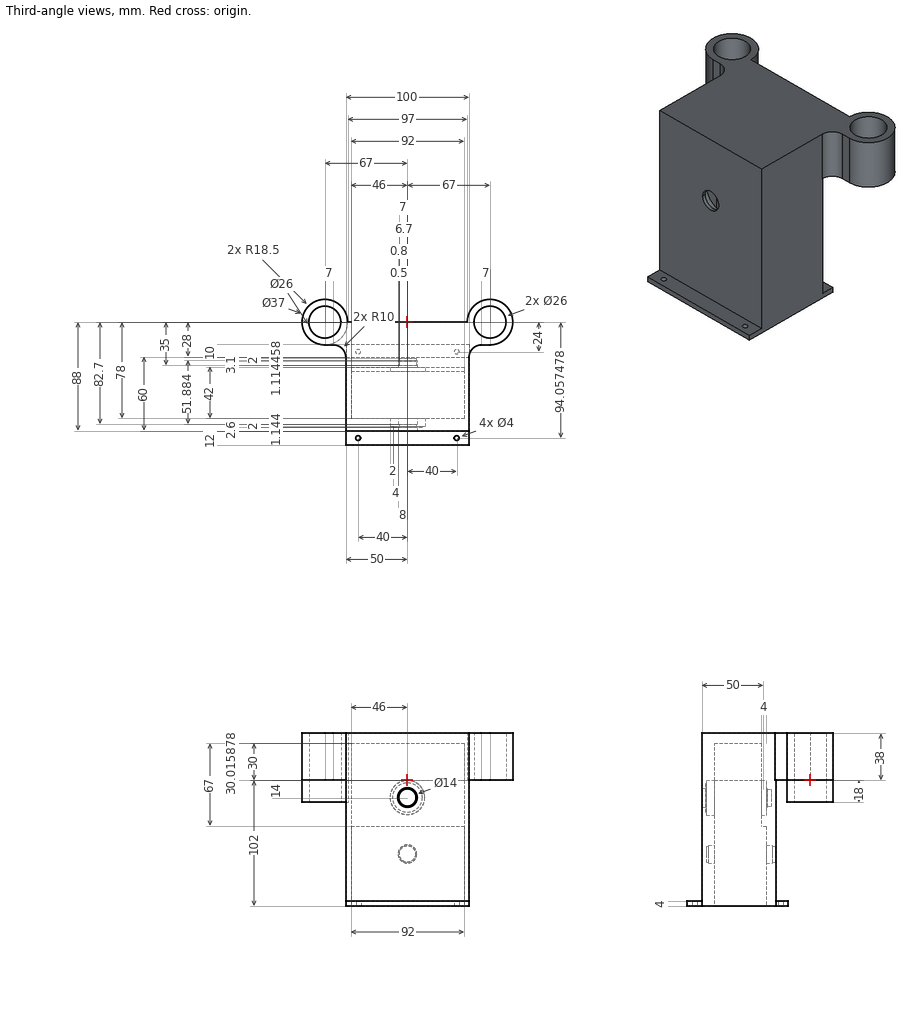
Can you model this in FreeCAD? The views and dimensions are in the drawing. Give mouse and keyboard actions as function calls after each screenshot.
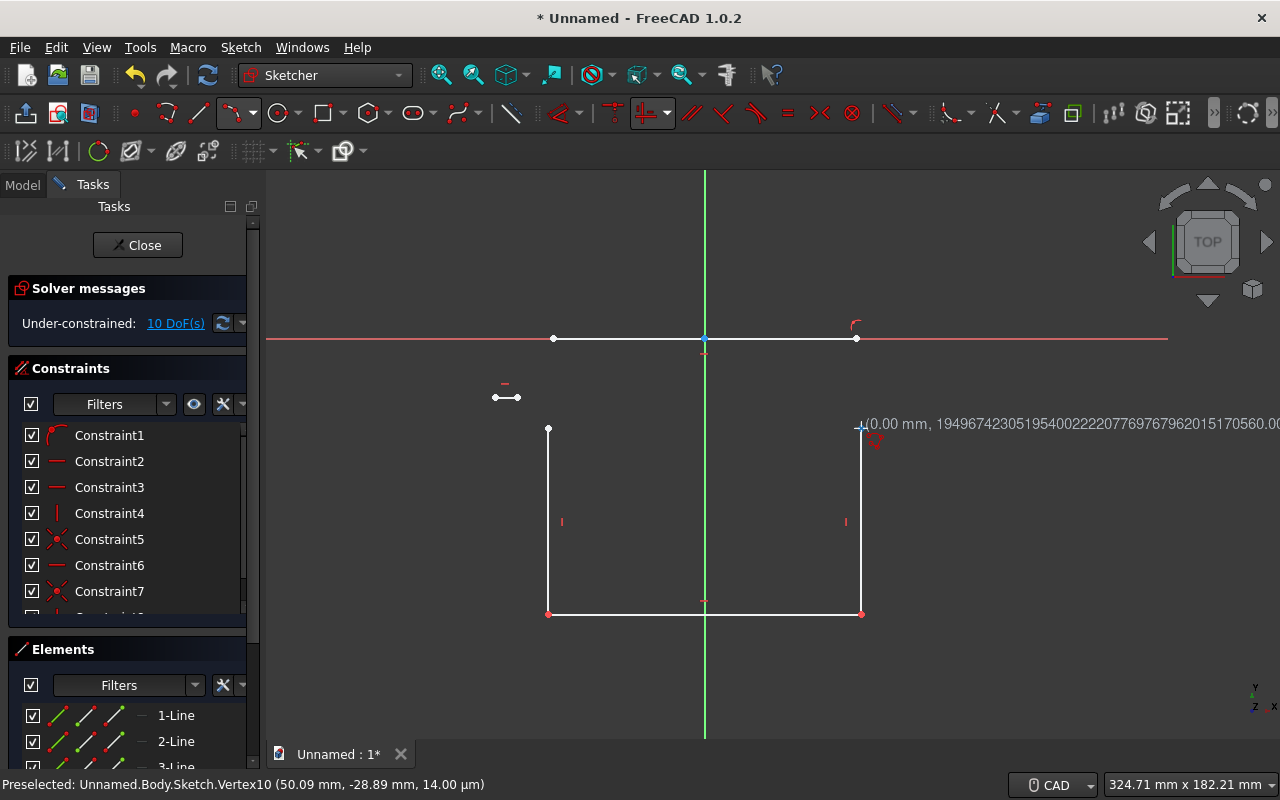
key(g)
key(l)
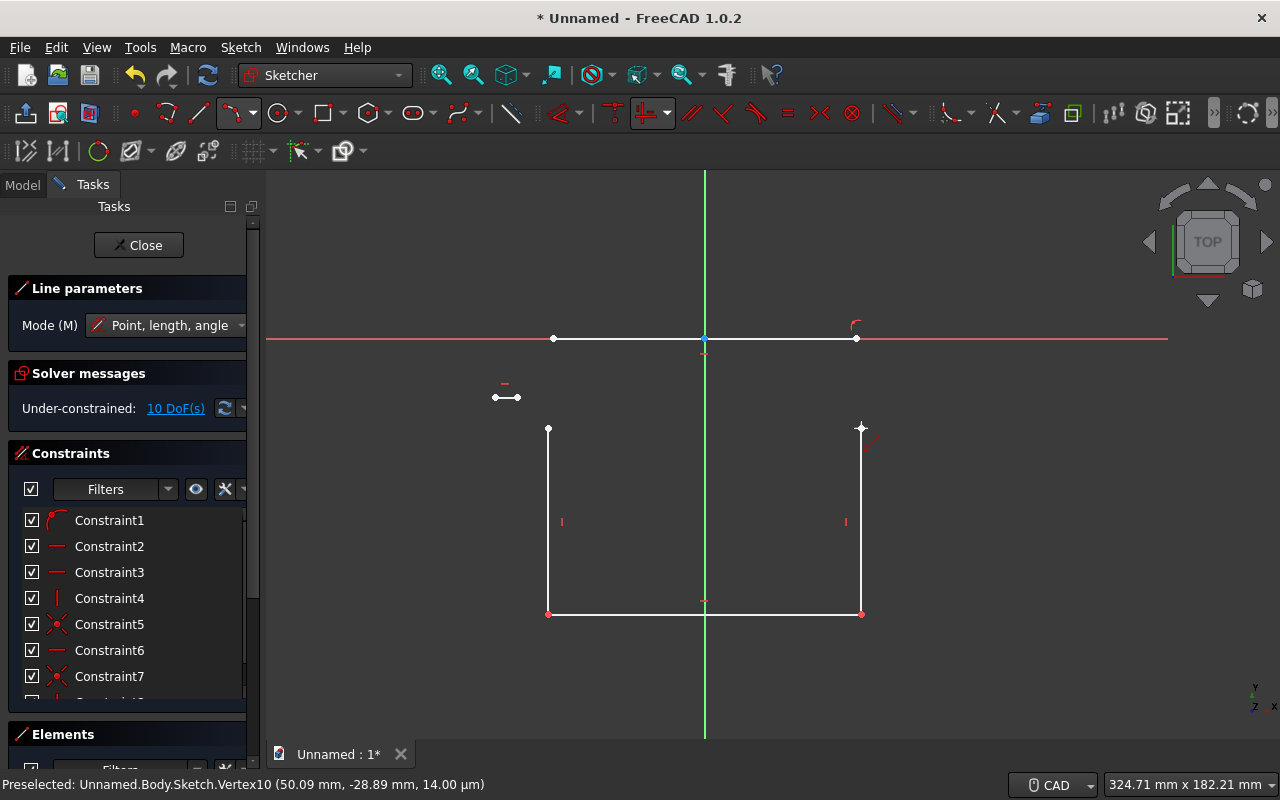
click(892, 397)
click(914, 397)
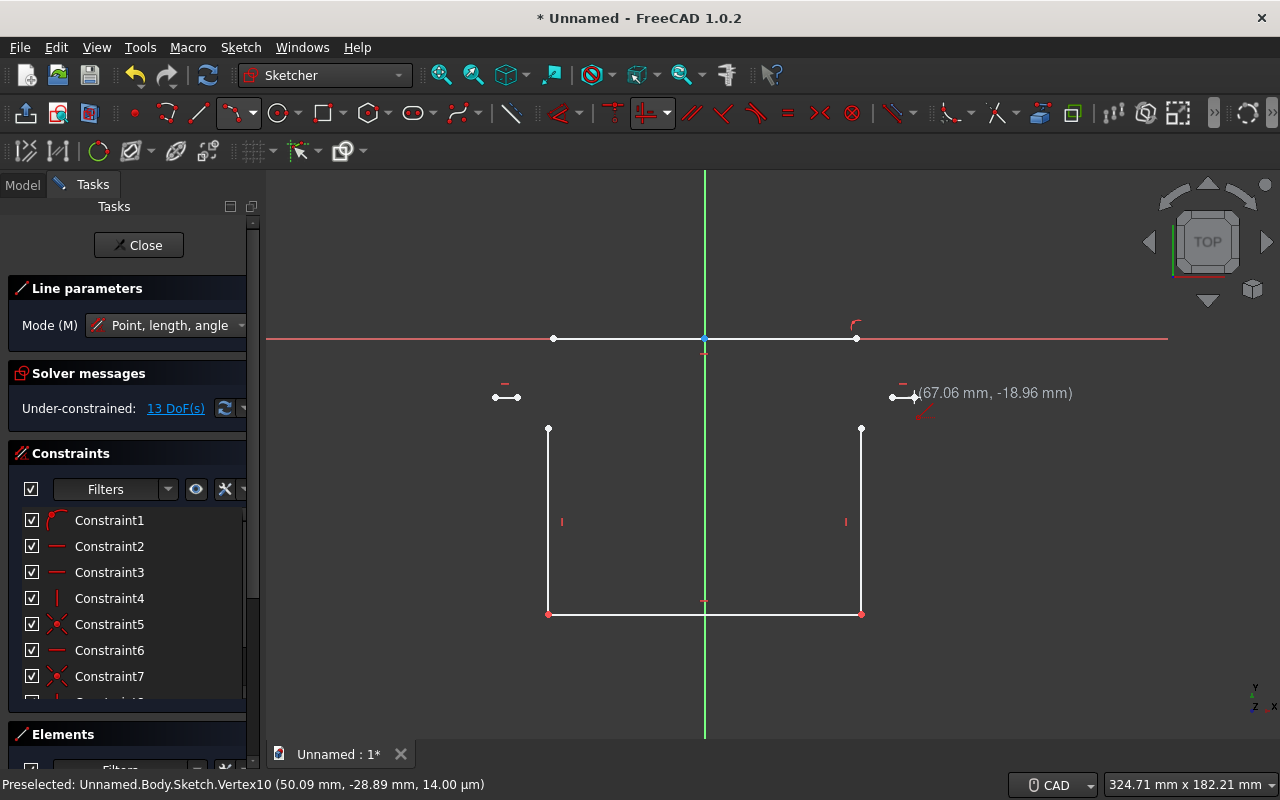
key(g)
key(3)
key(a)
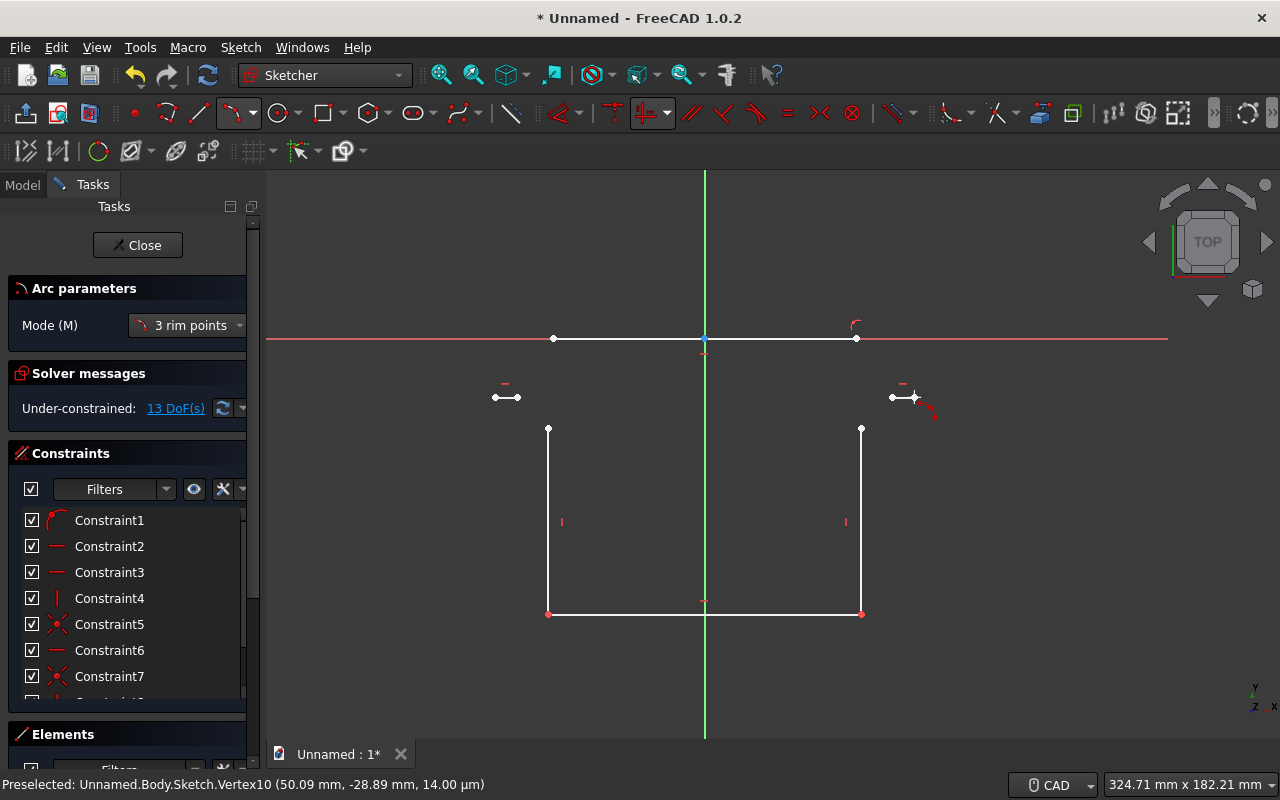
click(553, 348)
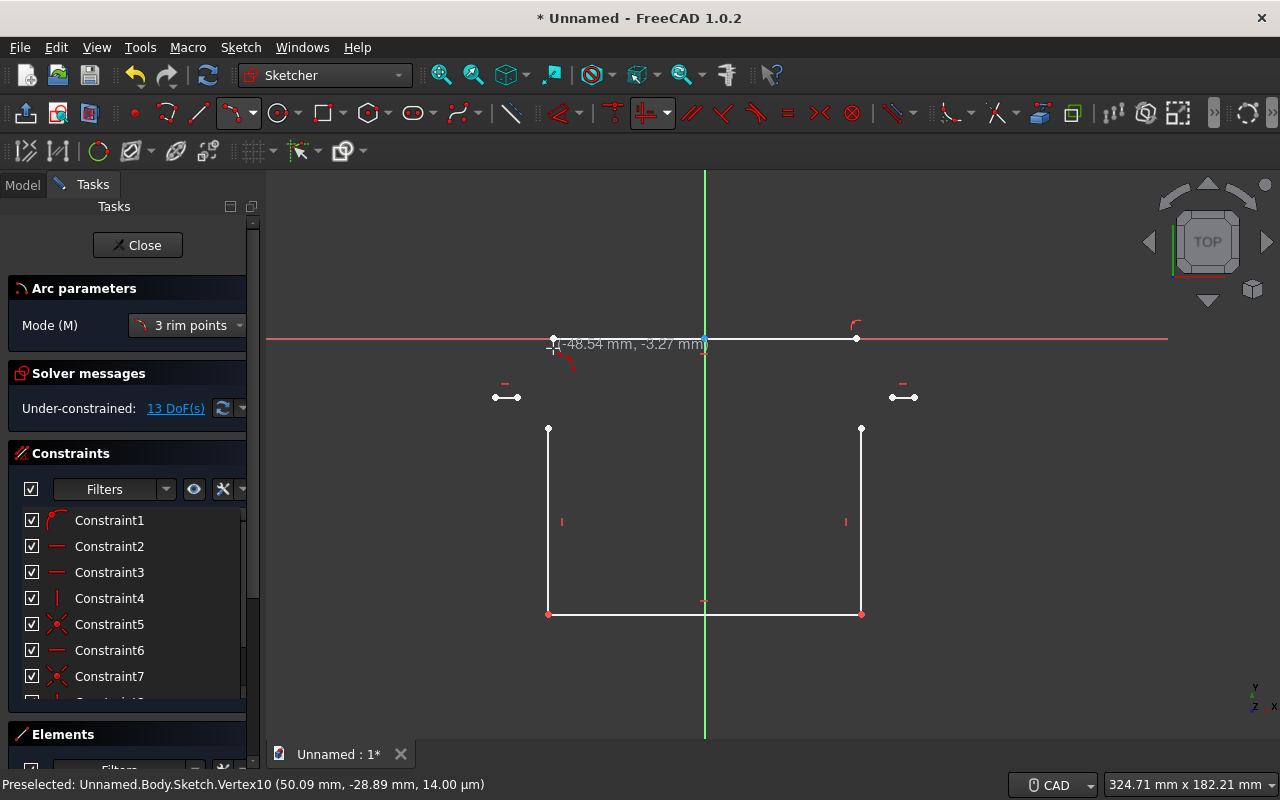
scroll(495, 397, up, 2)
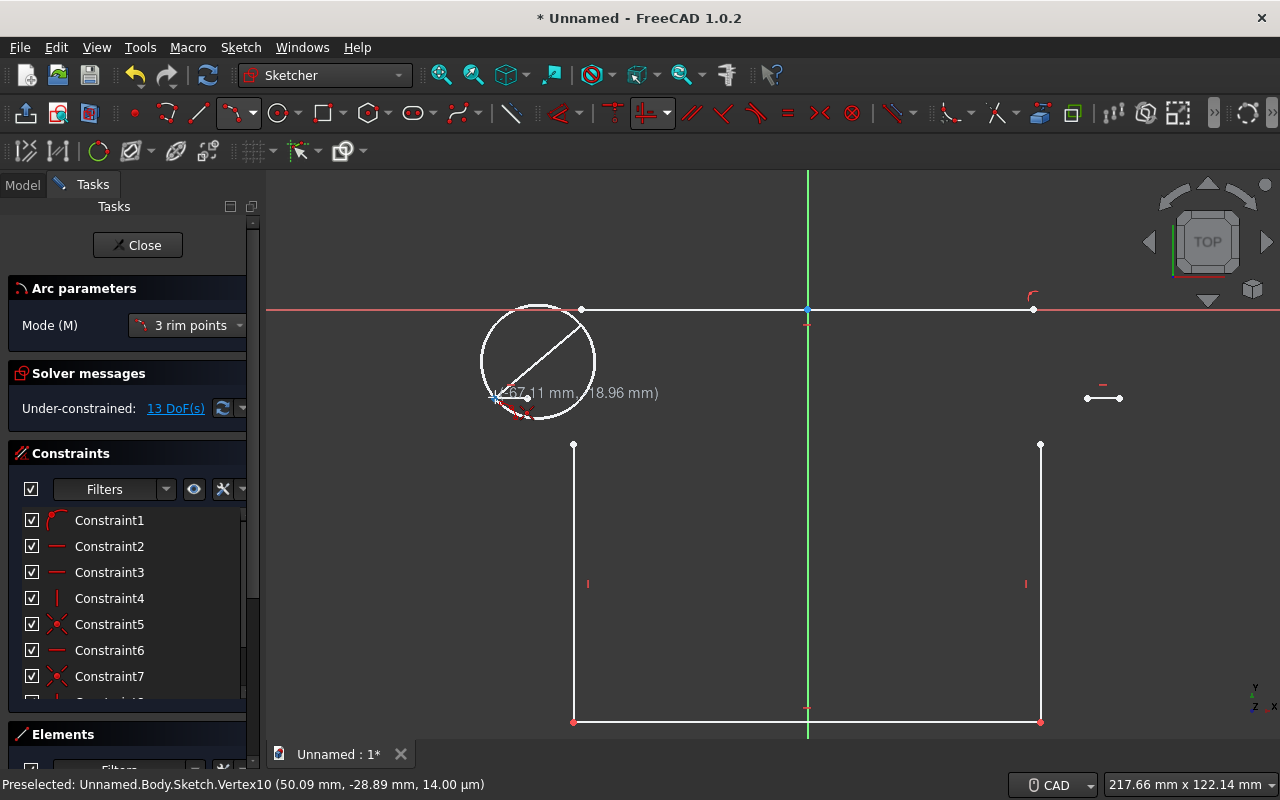
click(495, 398)
click(434, 249)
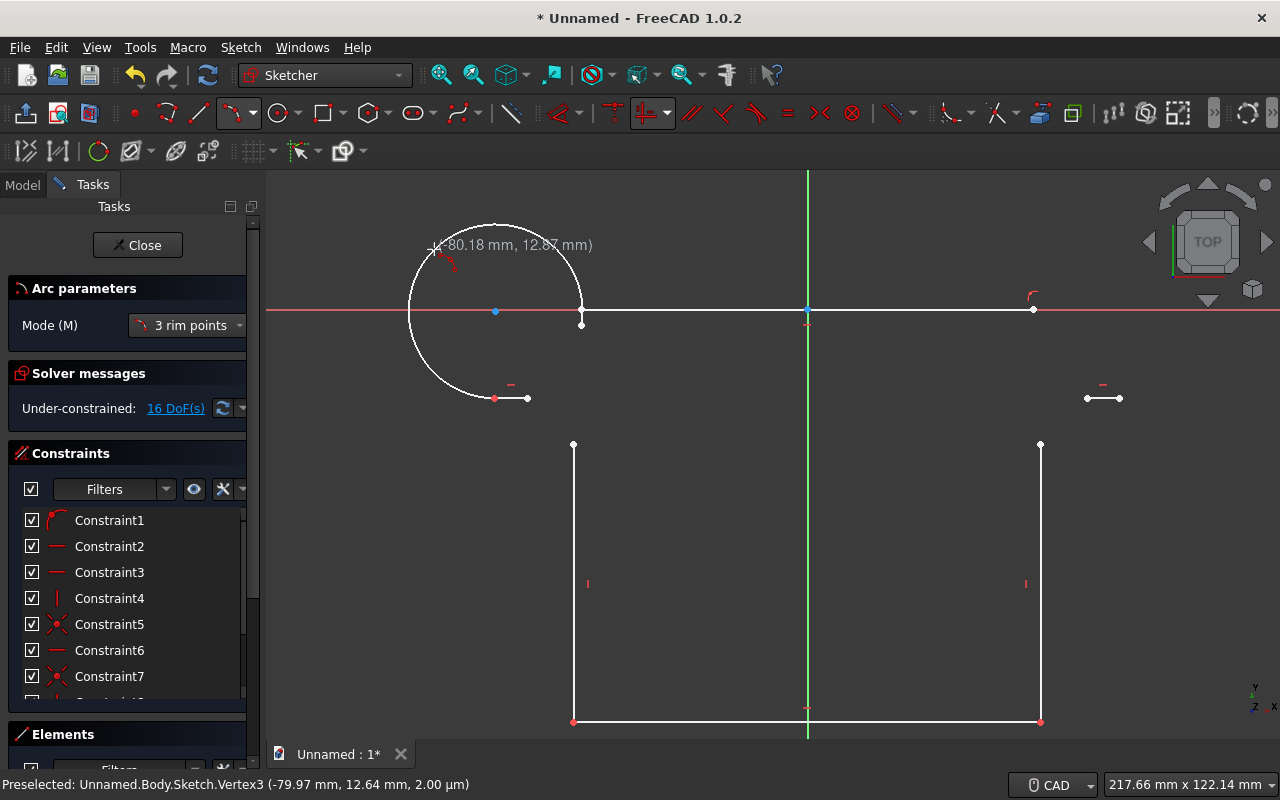
click(528, 398)
click(574, 445)
click(561, 410)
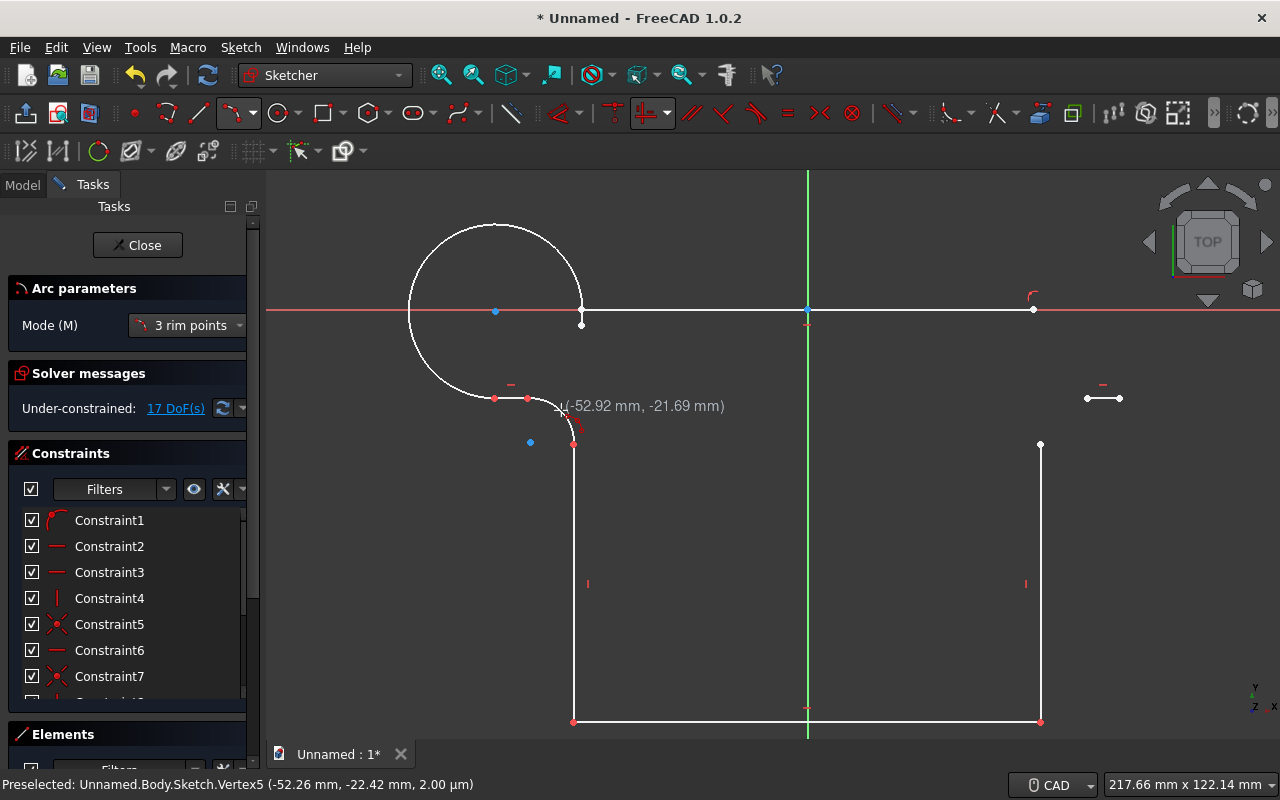
click(1041, 445)
click(1087, 398)
click(1054, 410)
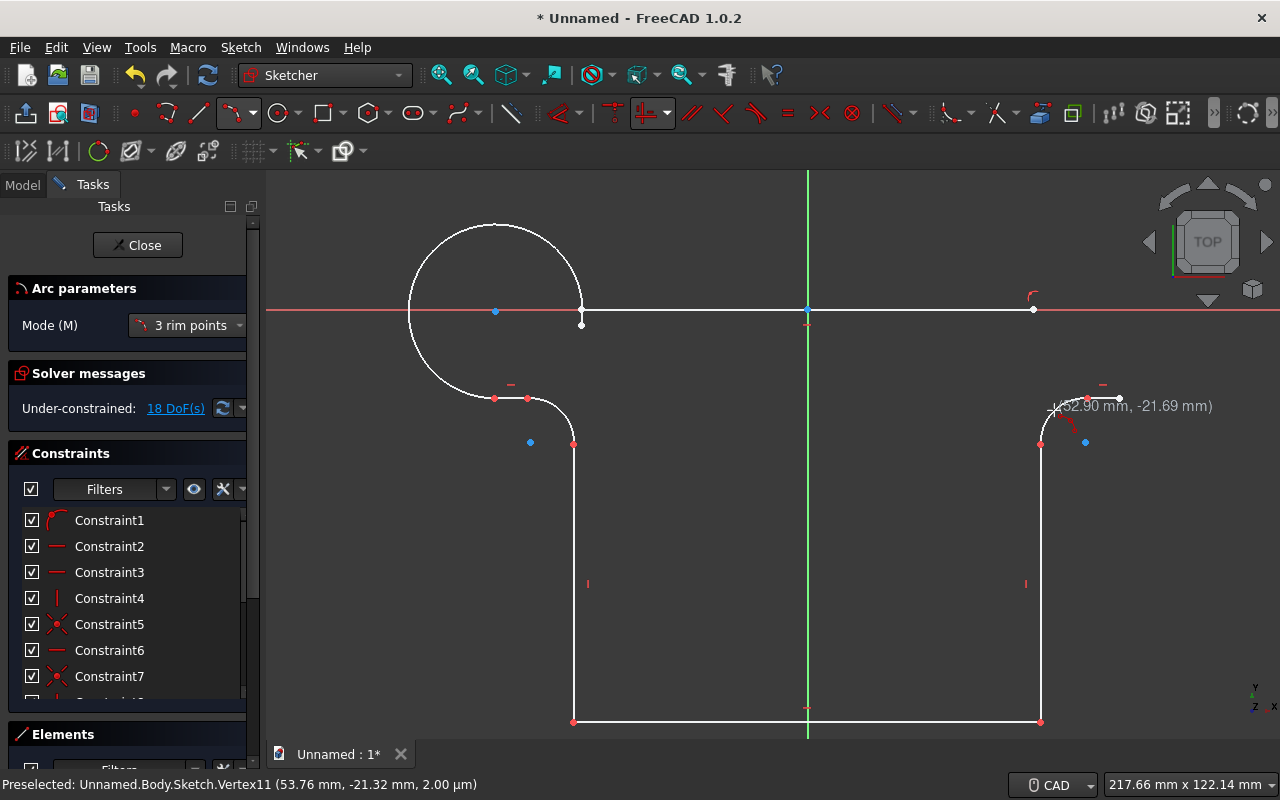
scroll(294, 319, down, 1)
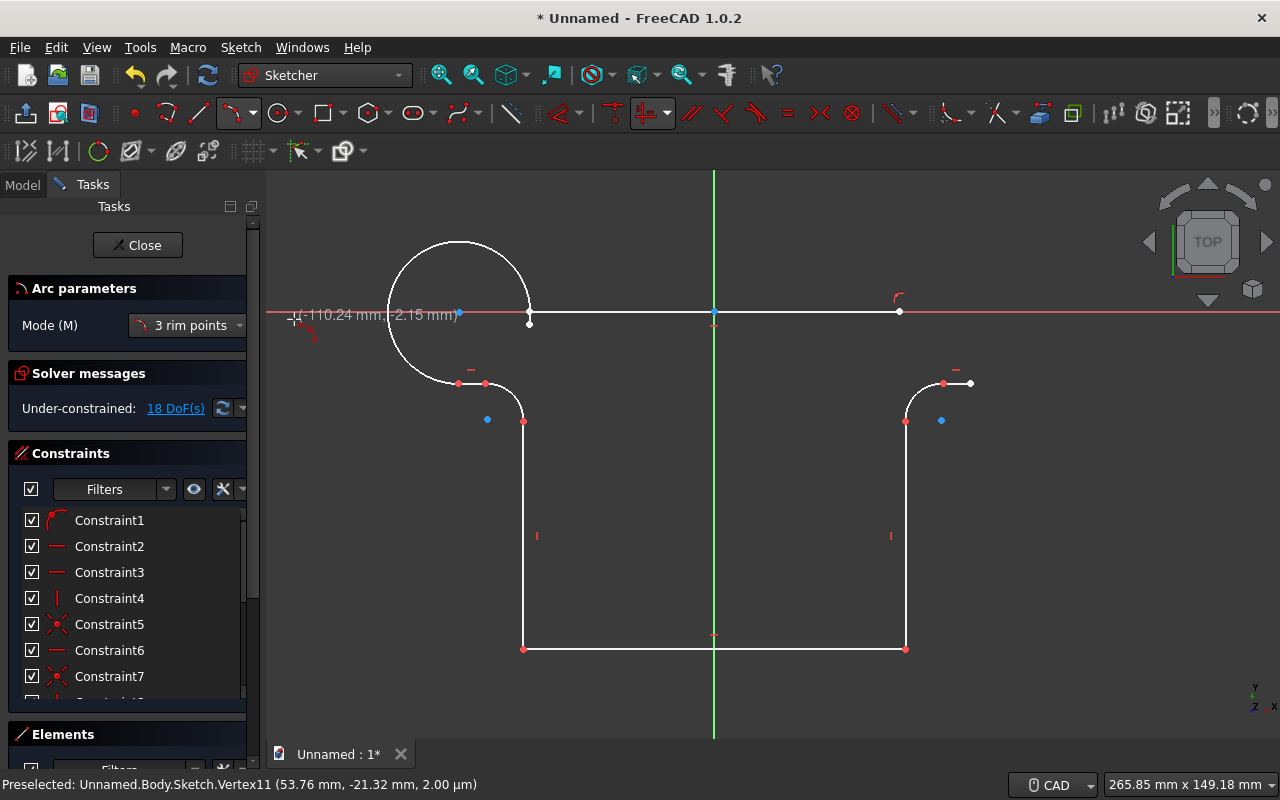
click(970, 384)
click(899, 312)
click(1020, 262)